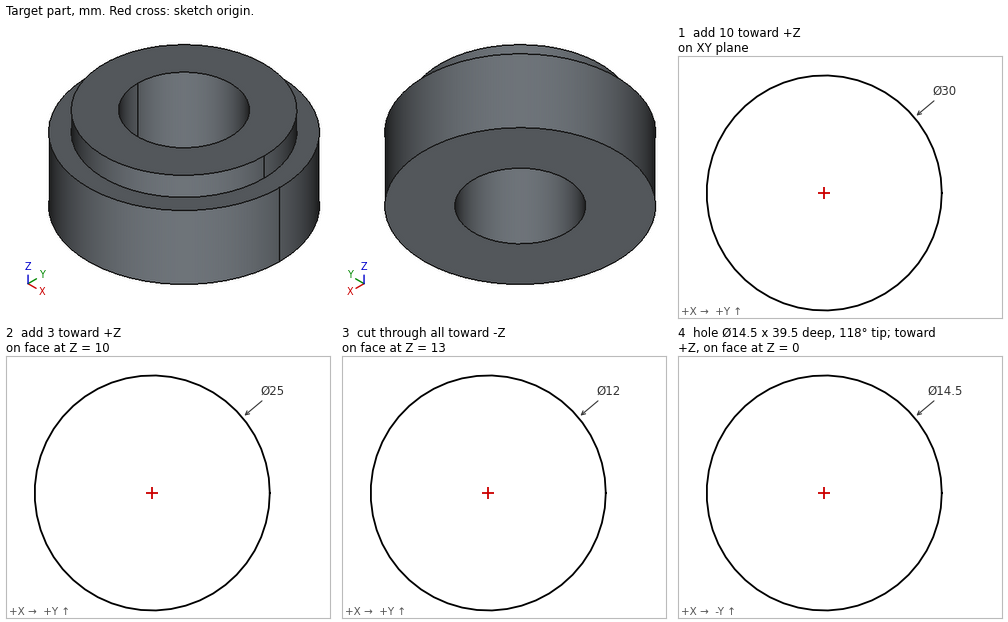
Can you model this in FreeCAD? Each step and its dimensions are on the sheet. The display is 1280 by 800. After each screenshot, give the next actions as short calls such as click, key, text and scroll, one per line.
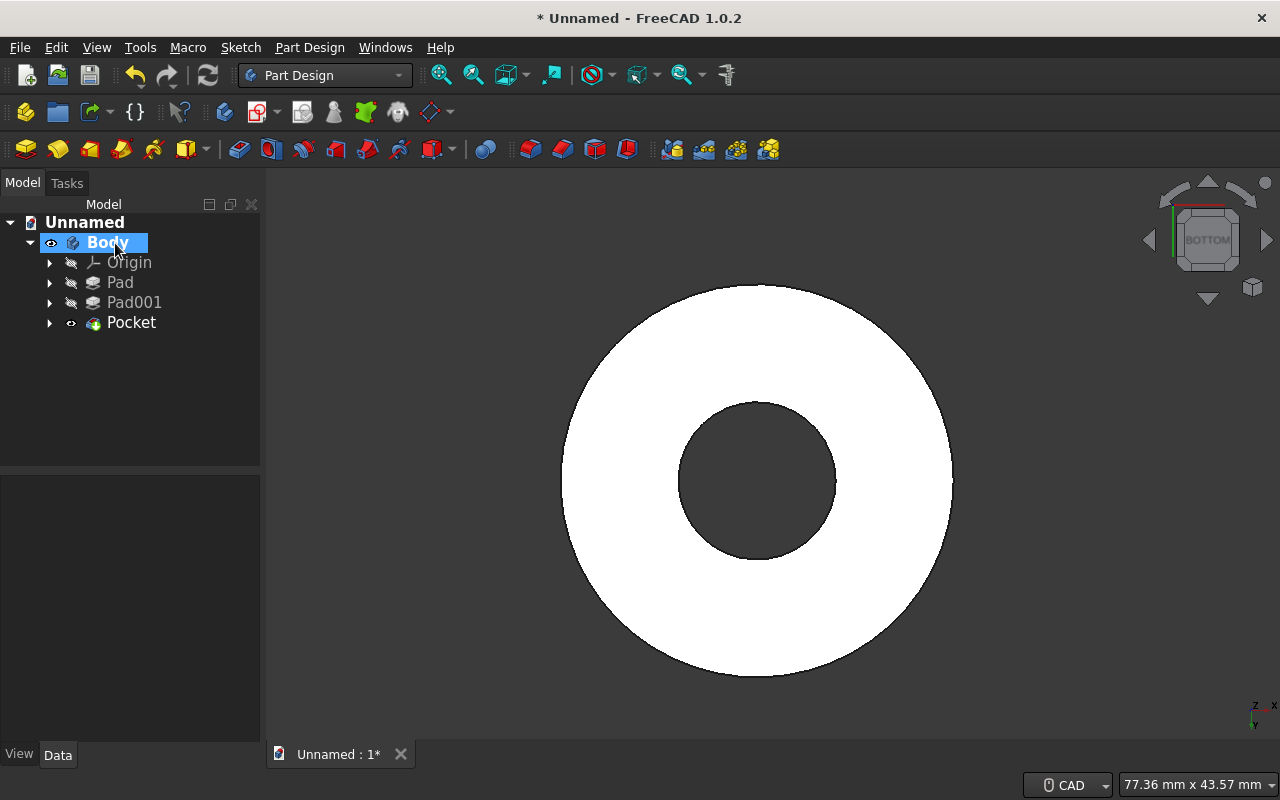
click(869, 424)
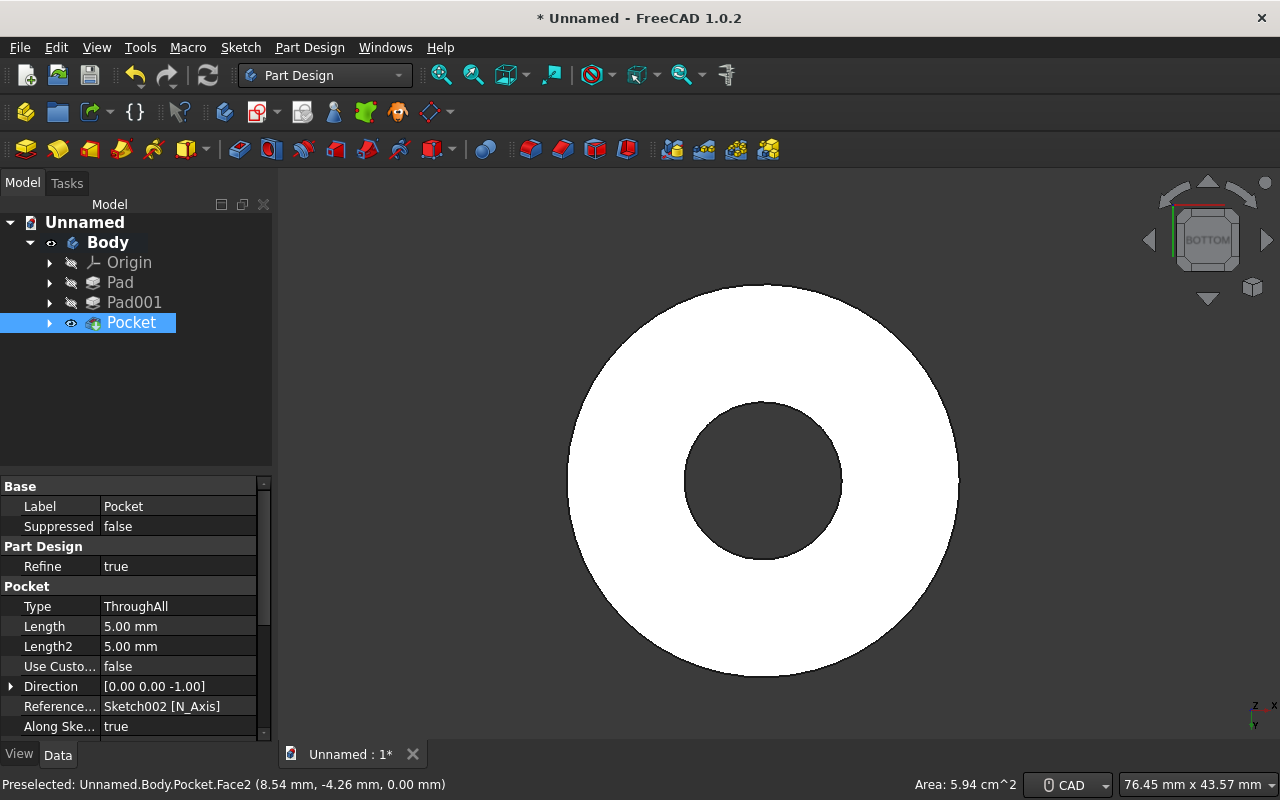
click(258, 112)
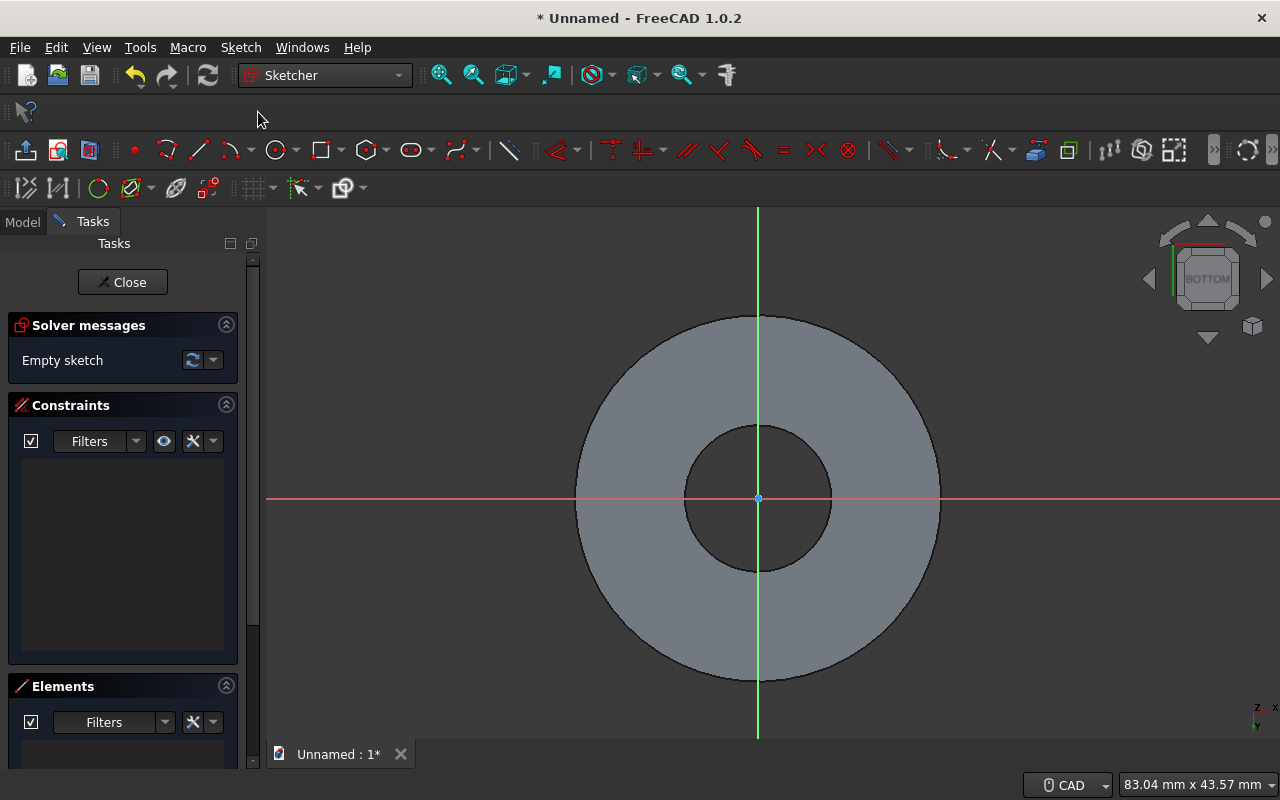
scroll(823, 530, up, 3)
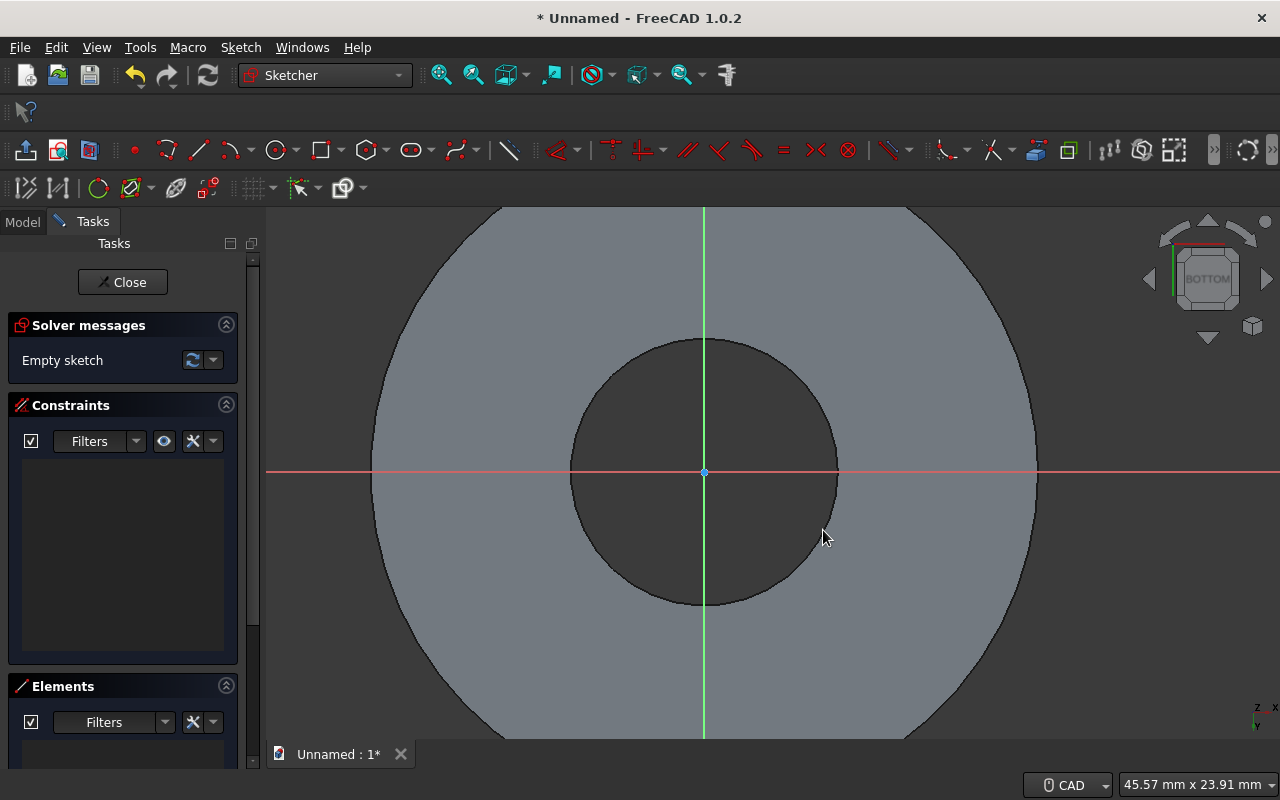
click(276, 150)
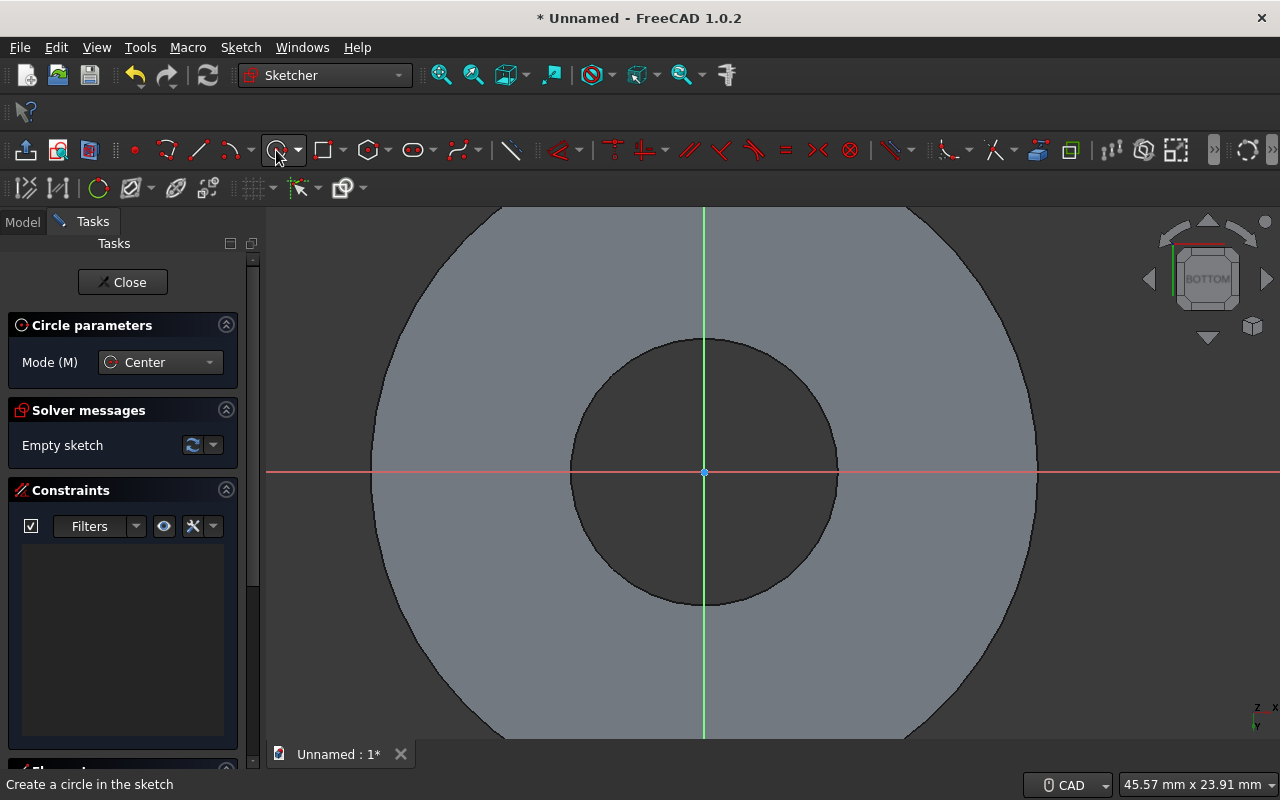
click(704, 472)
click(818, 358)
key(Escape)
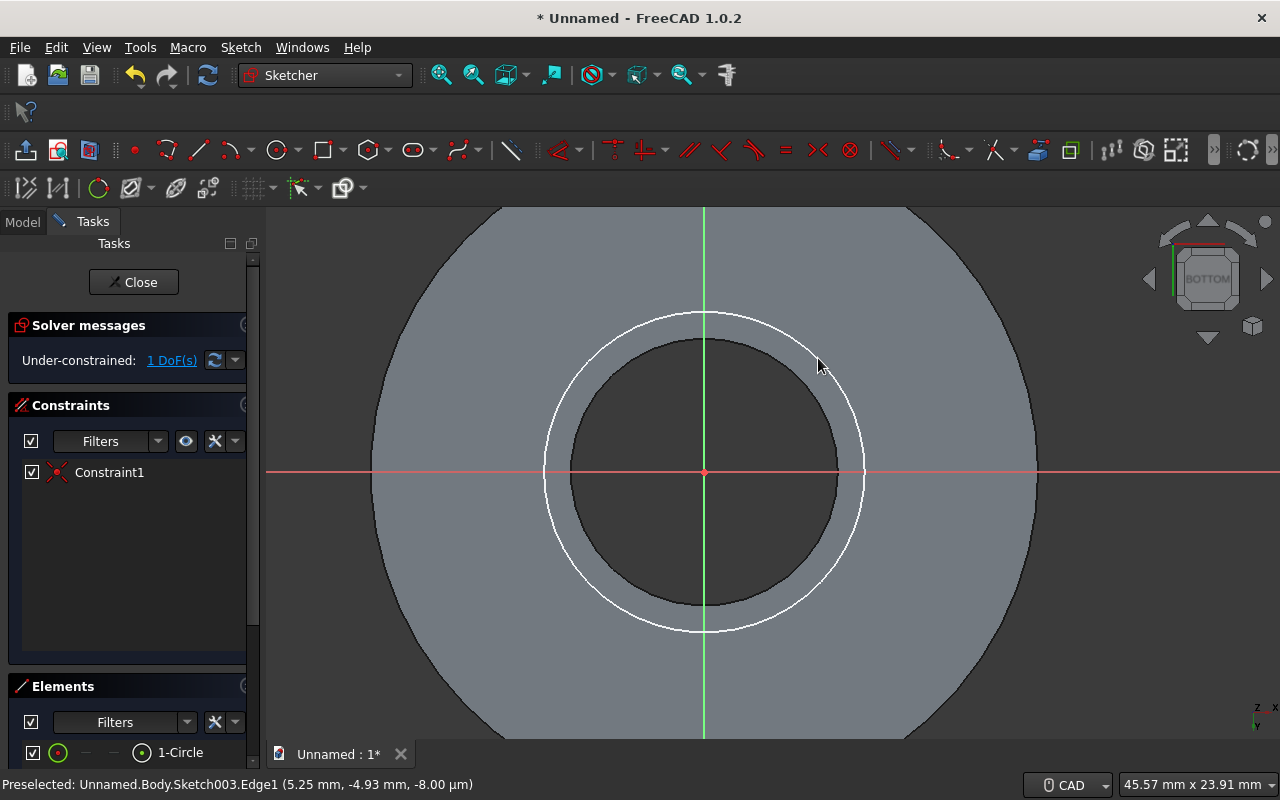
click(558, 150)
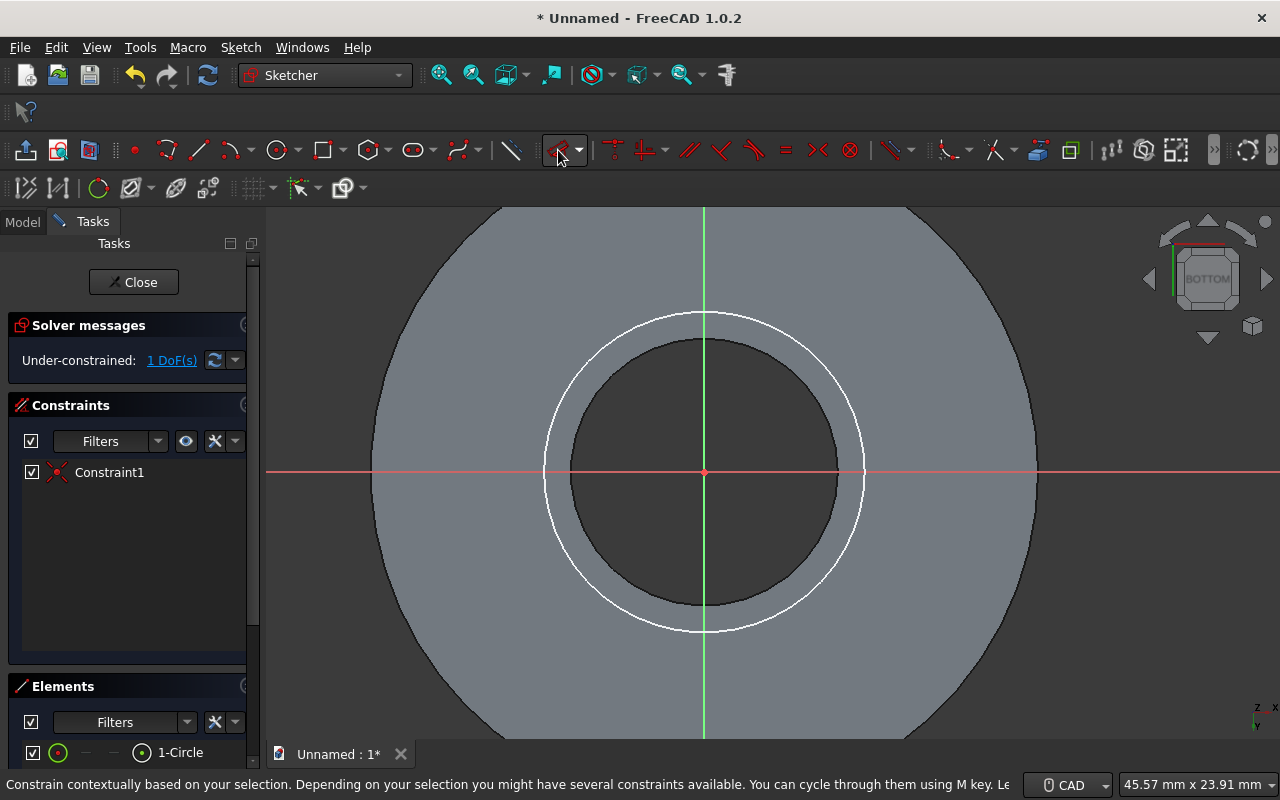
click(817, 358)
click(839, 335)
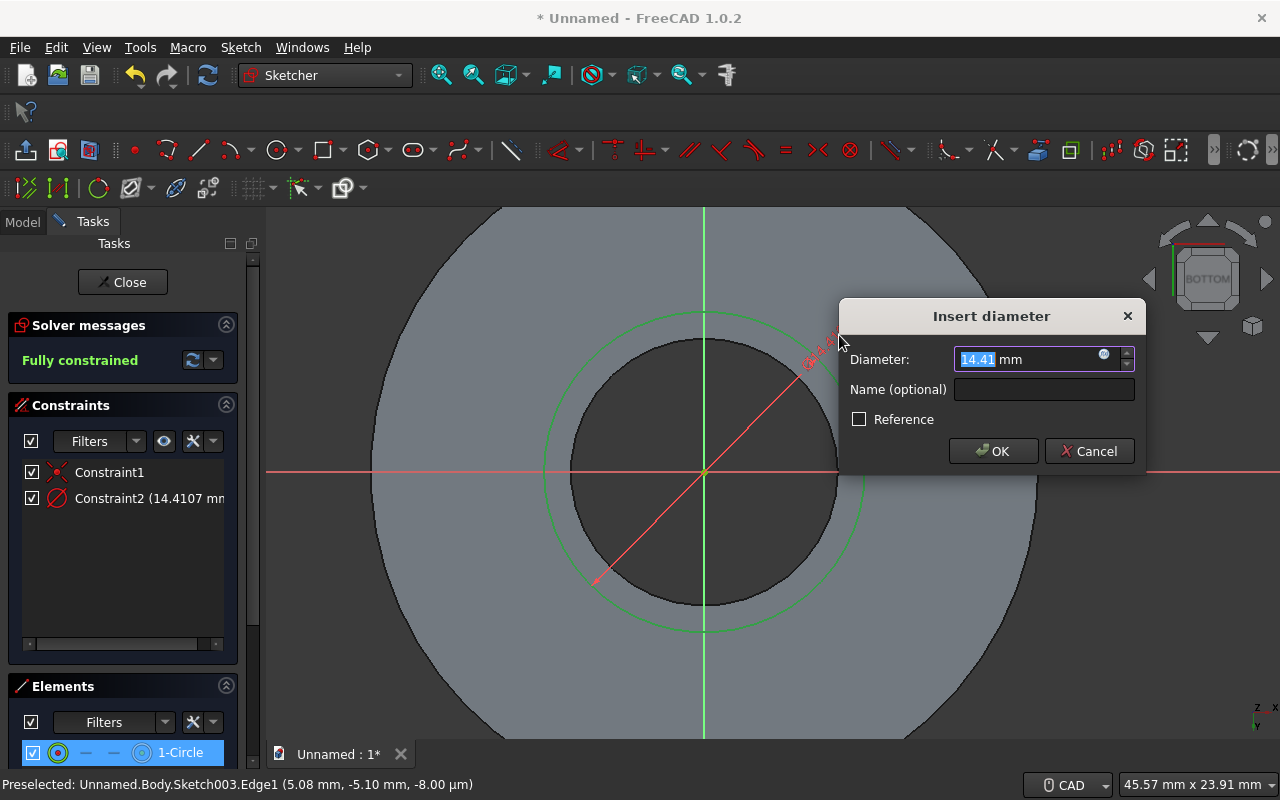
text(14.5)
key(Return)
key(Escape)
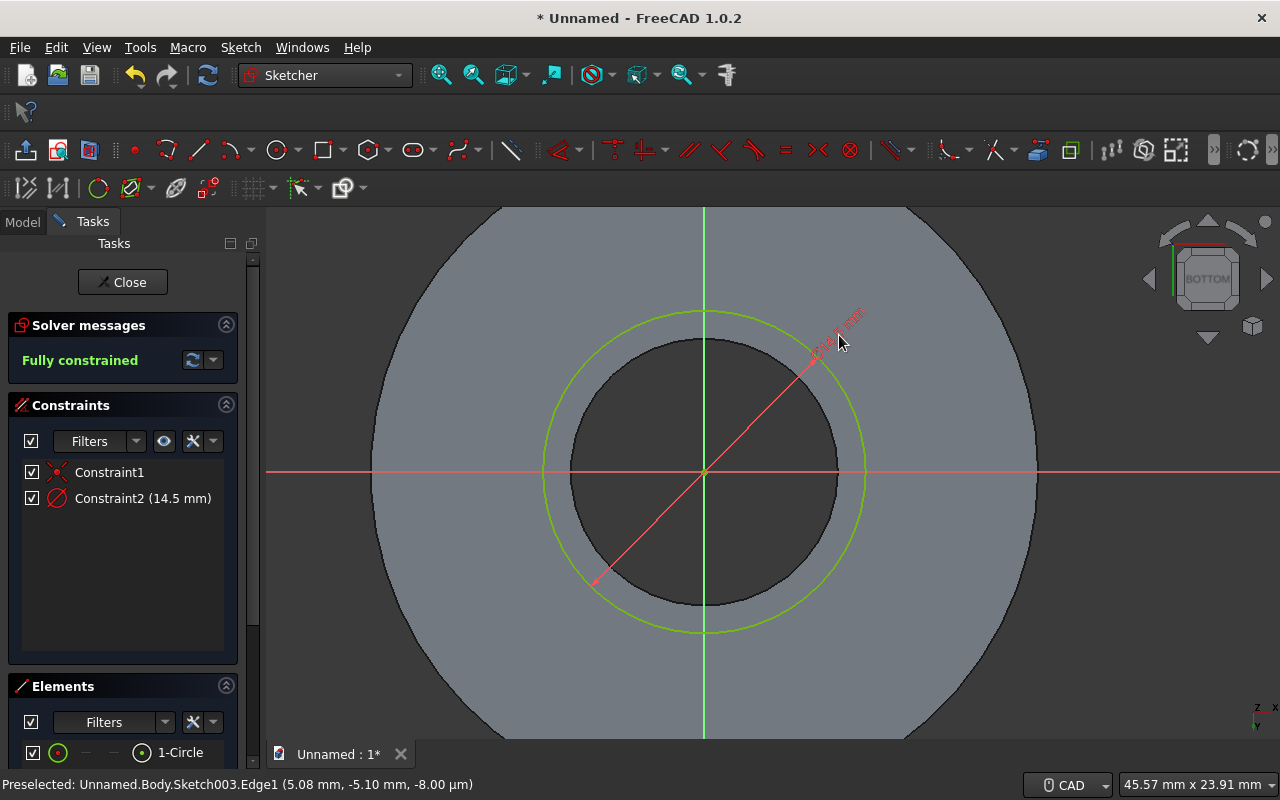
click(123, 282)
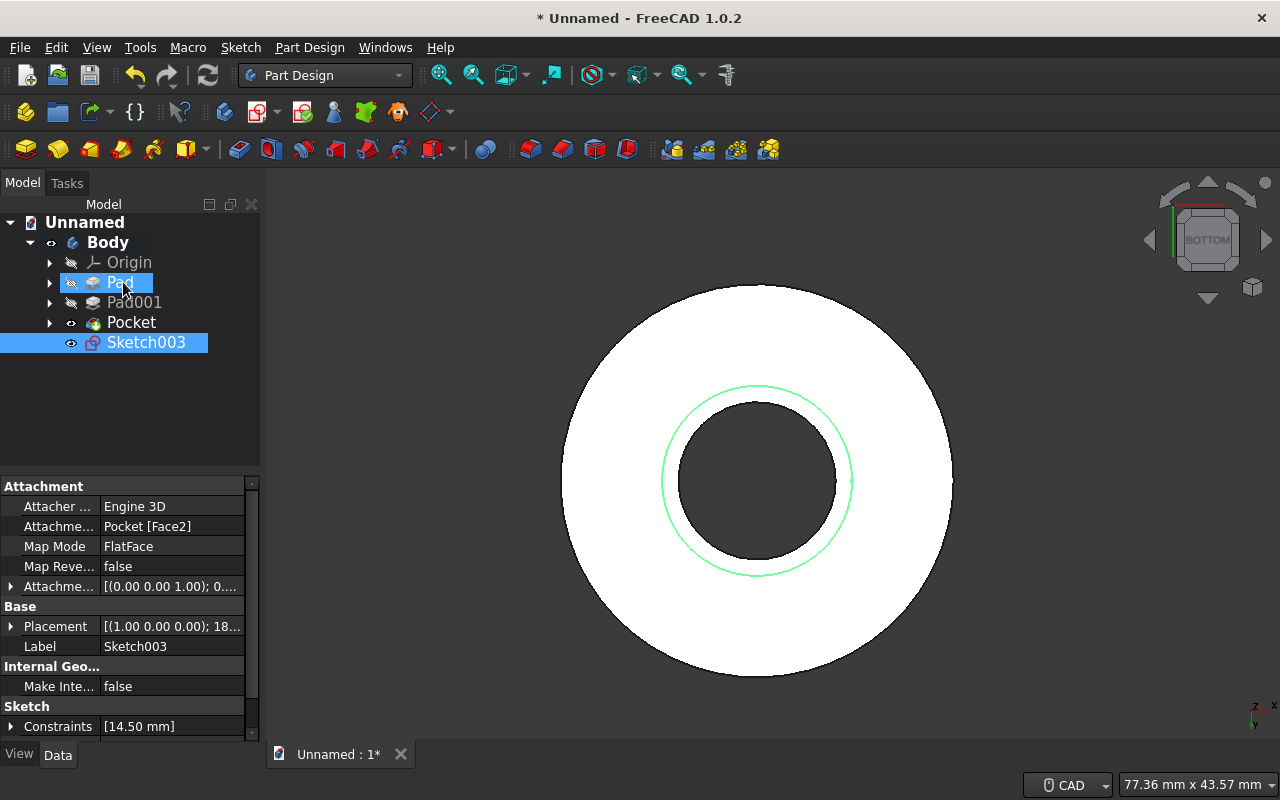
click(272, 150)